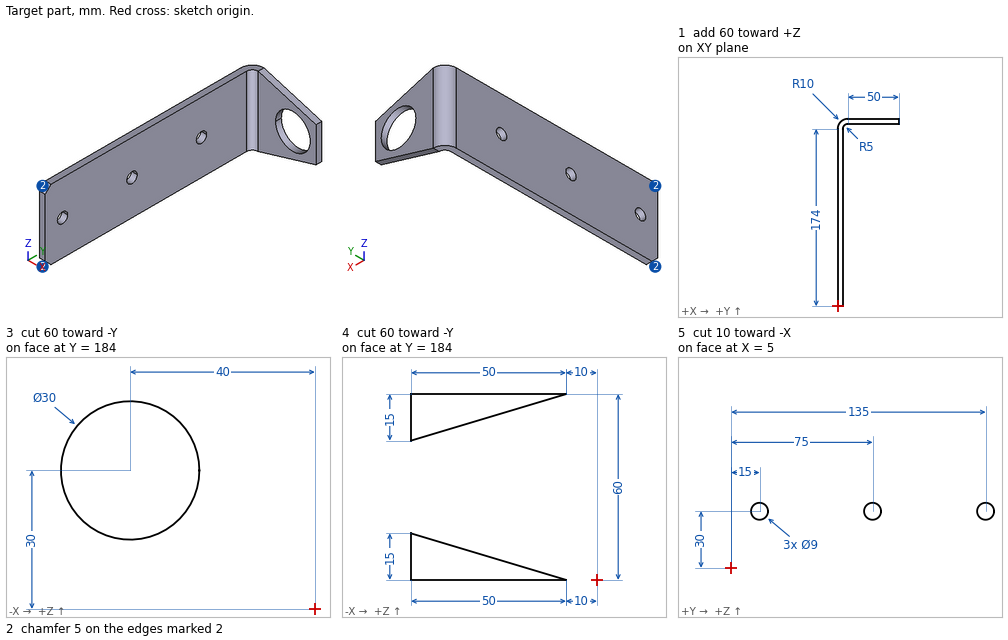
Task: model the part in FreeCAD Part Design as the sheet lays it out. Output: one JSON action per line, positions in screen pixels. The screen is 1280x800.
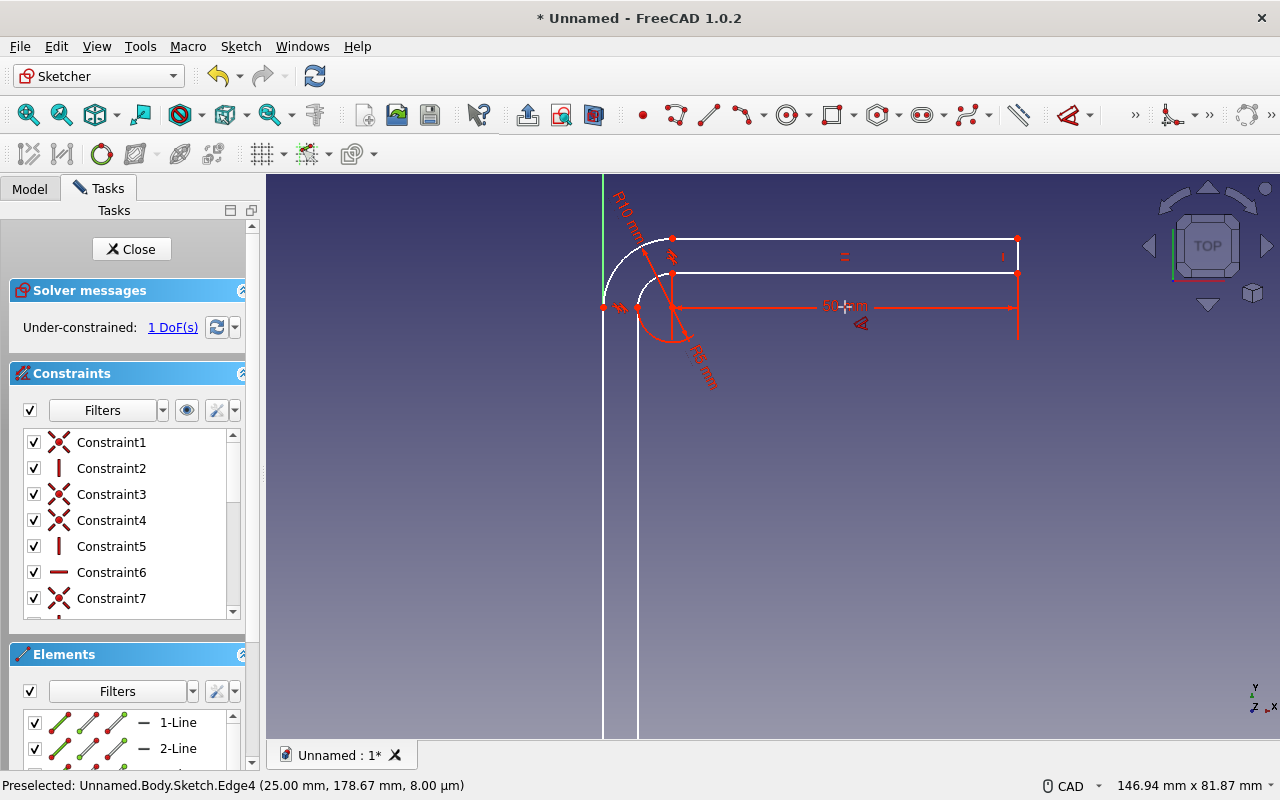
{"action": "left_click", "coordinate": [603, 668]}
{"action": "left_click", "coordinate": [569, 509]}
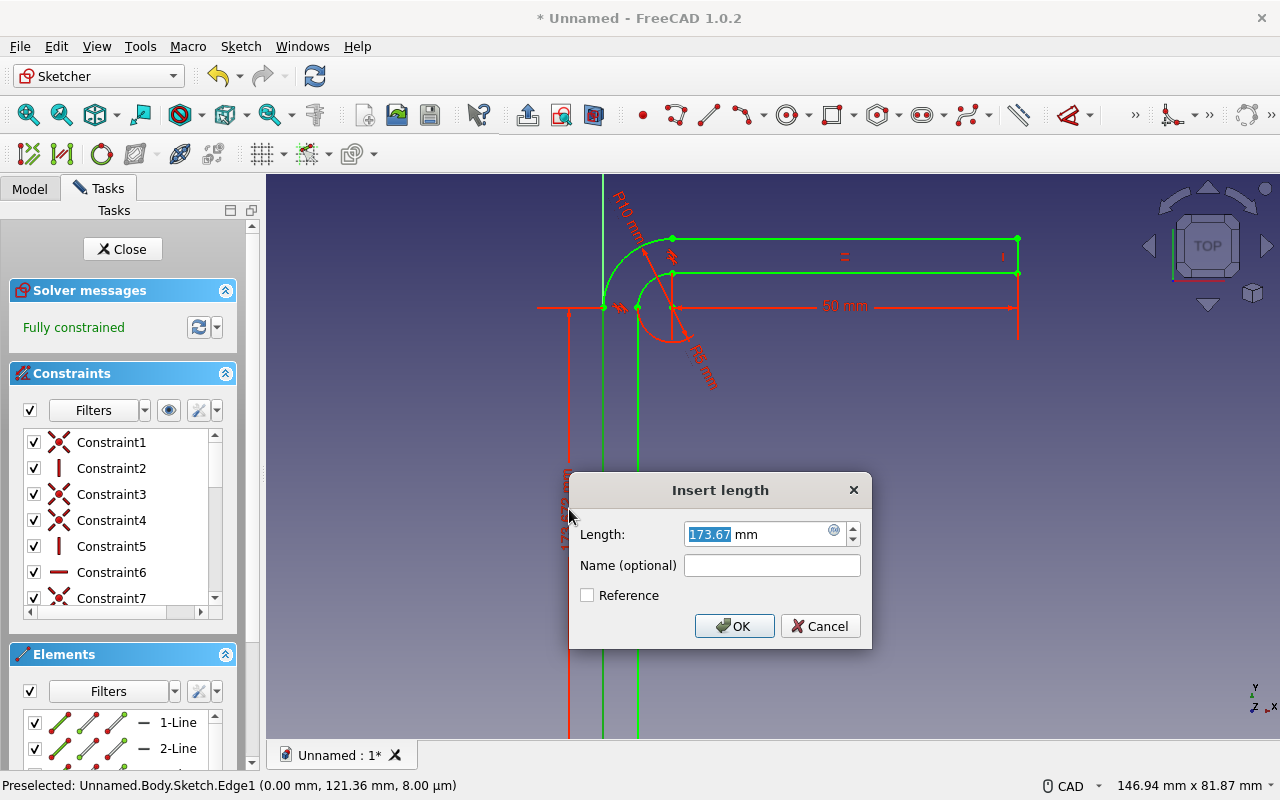
{"action": "type", "text": "174"}
{"action": "key", "text": "Return"}
{"action": "key", "text": "Escape"}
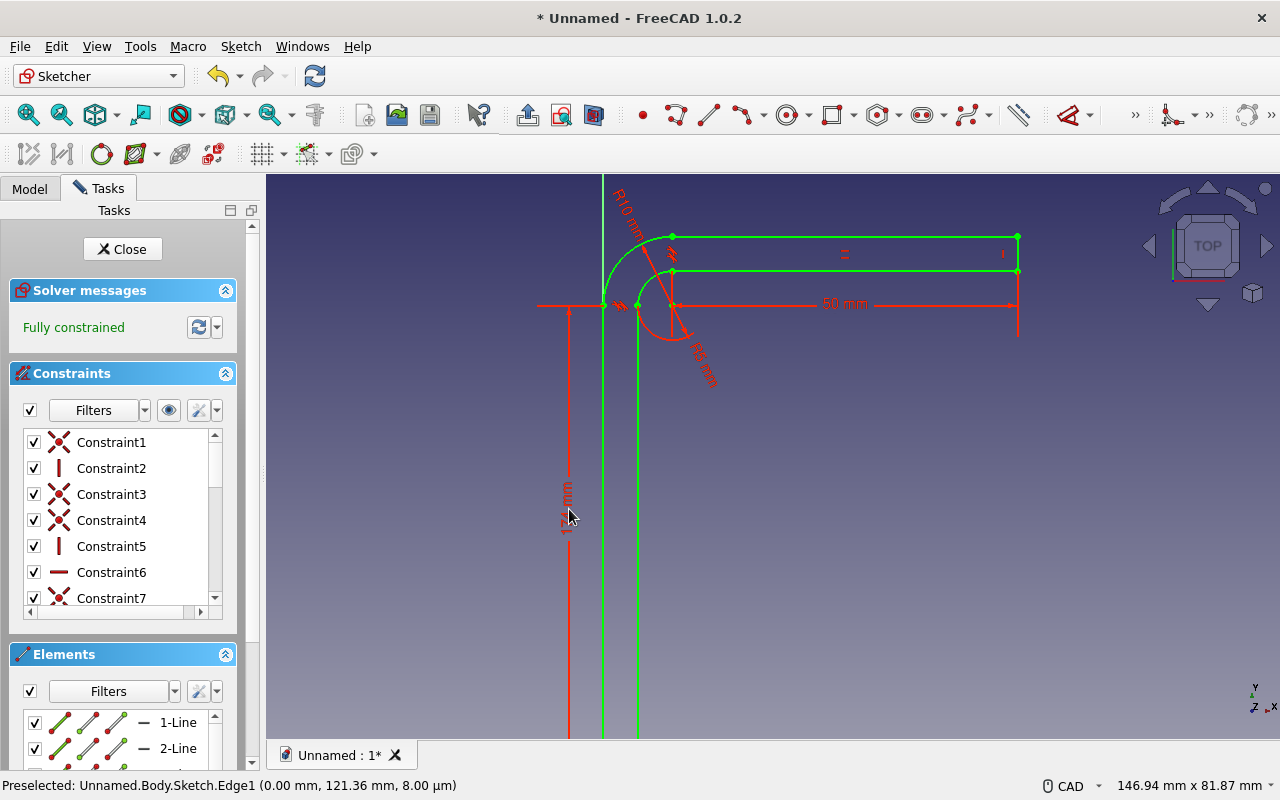
{"action": "left_click", "coordinate": [123, 249]}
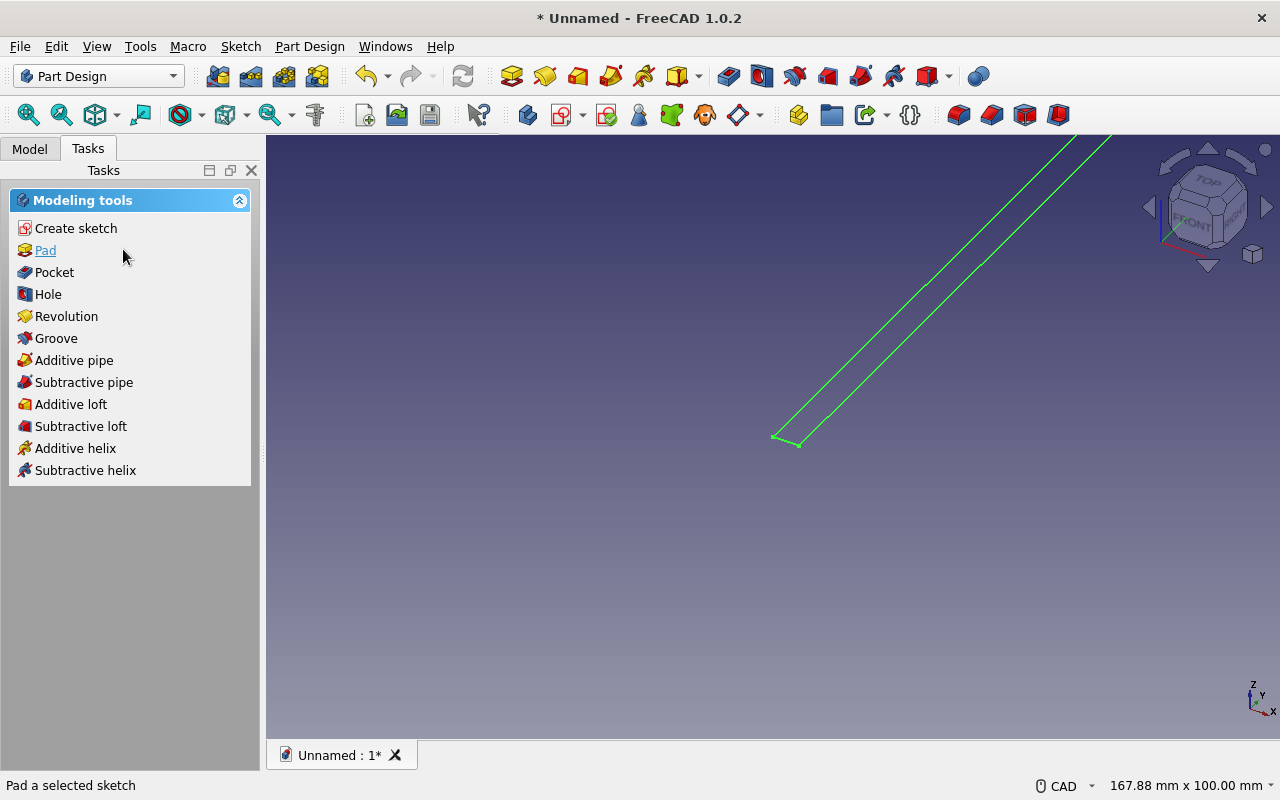
{"action": "left_click", "coordinate": [512, 76]}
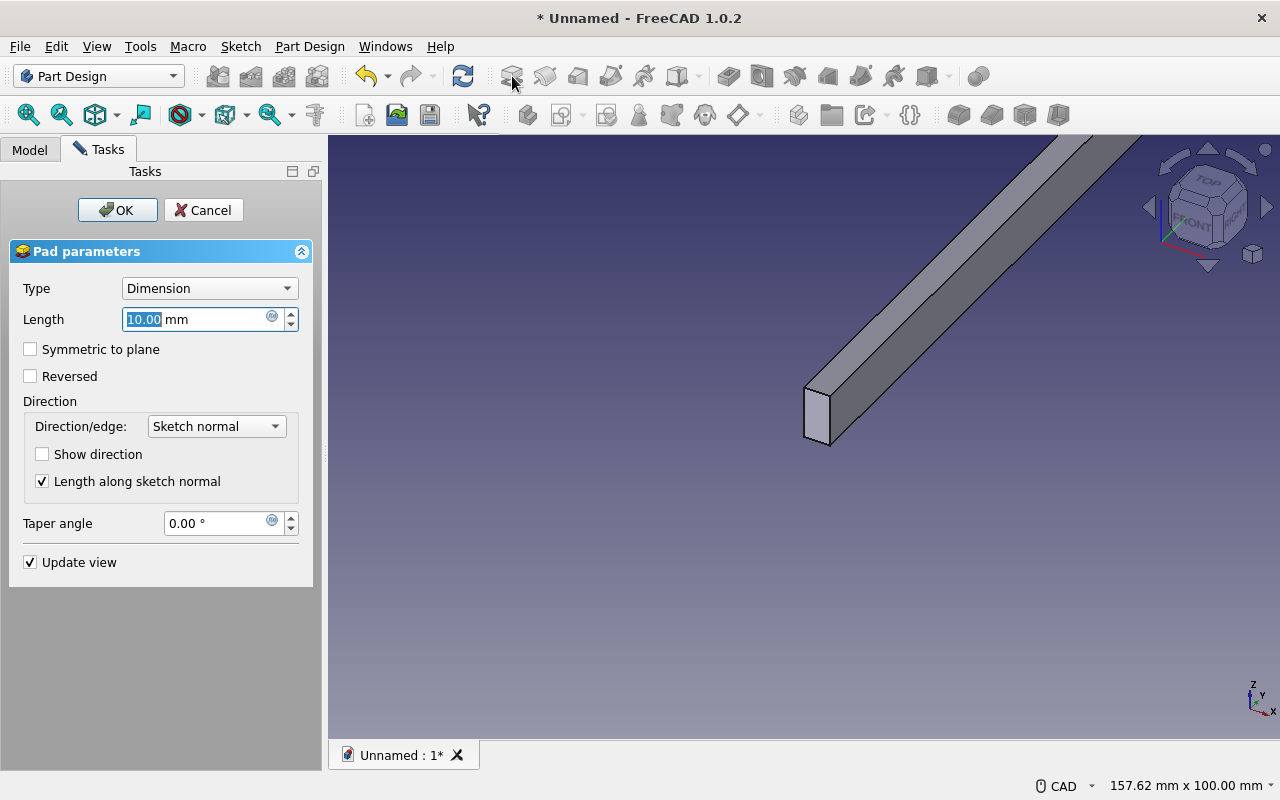
{"action": "type", "text": "60"}
{"action": "key", "text": "Tab"}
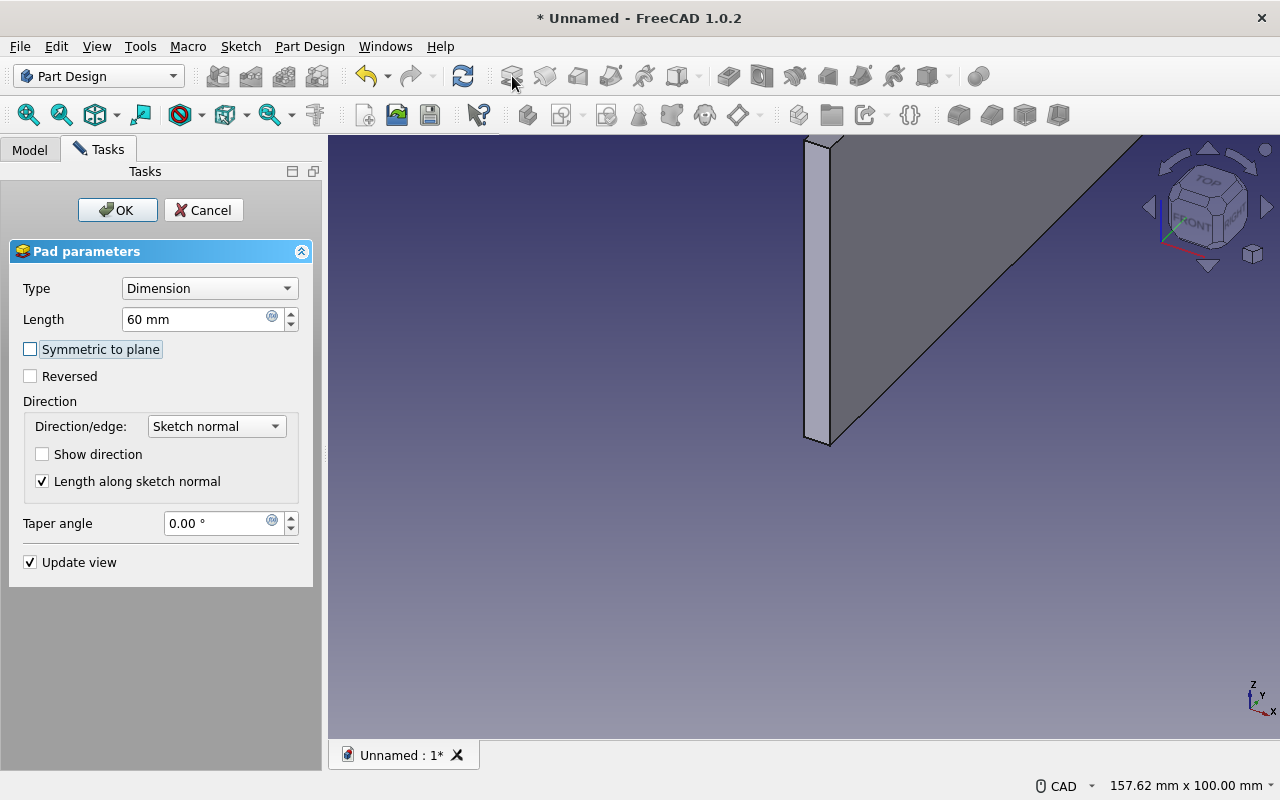
{"action": "left_click", "coordinate": [118, 210]}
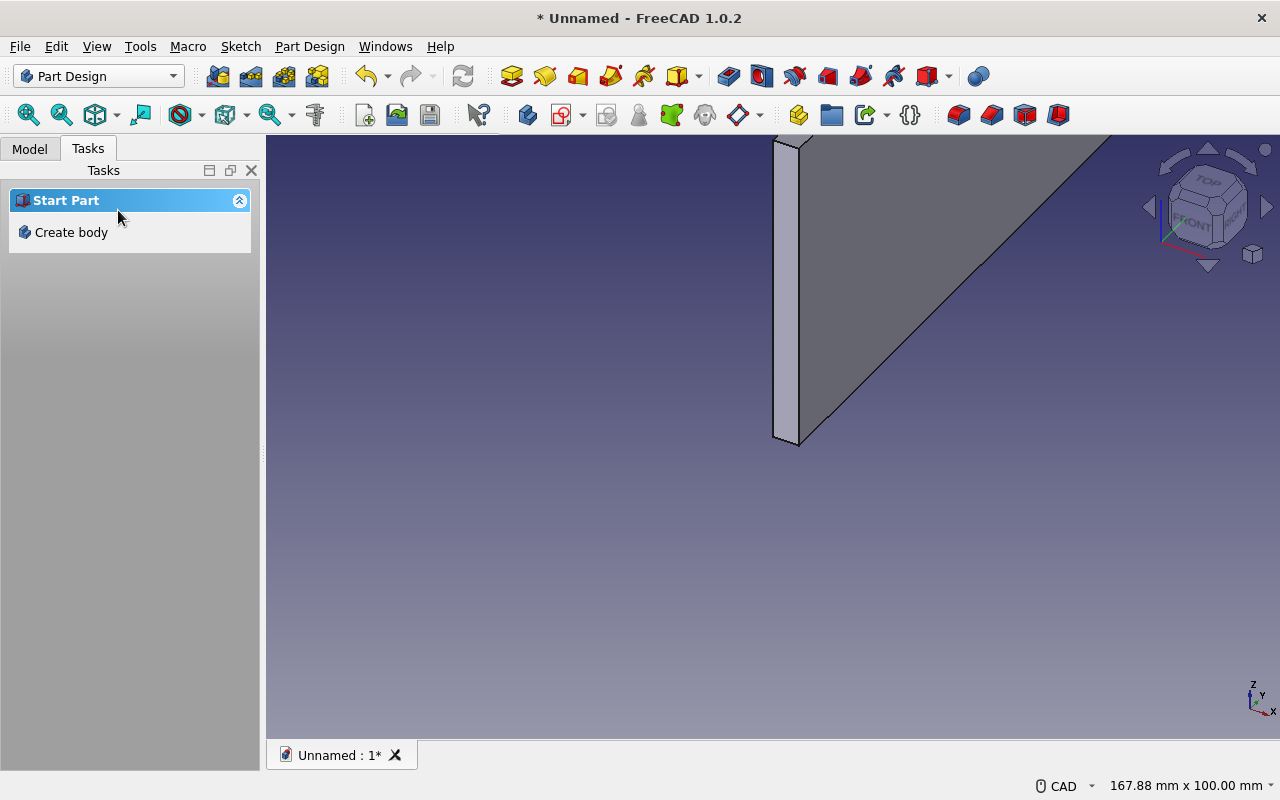
{"action": "key", "text": "v f"}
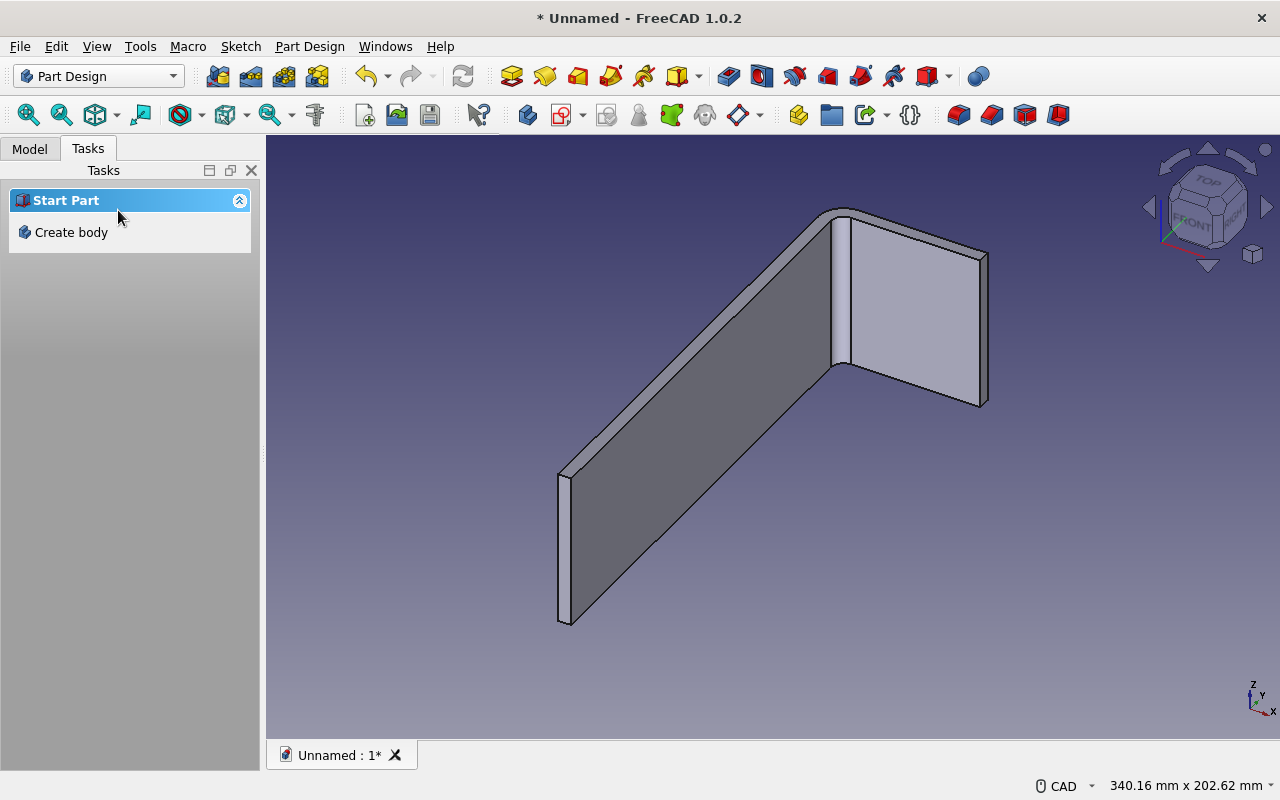
{"action": "left_click", "coordinate": [565, 475]}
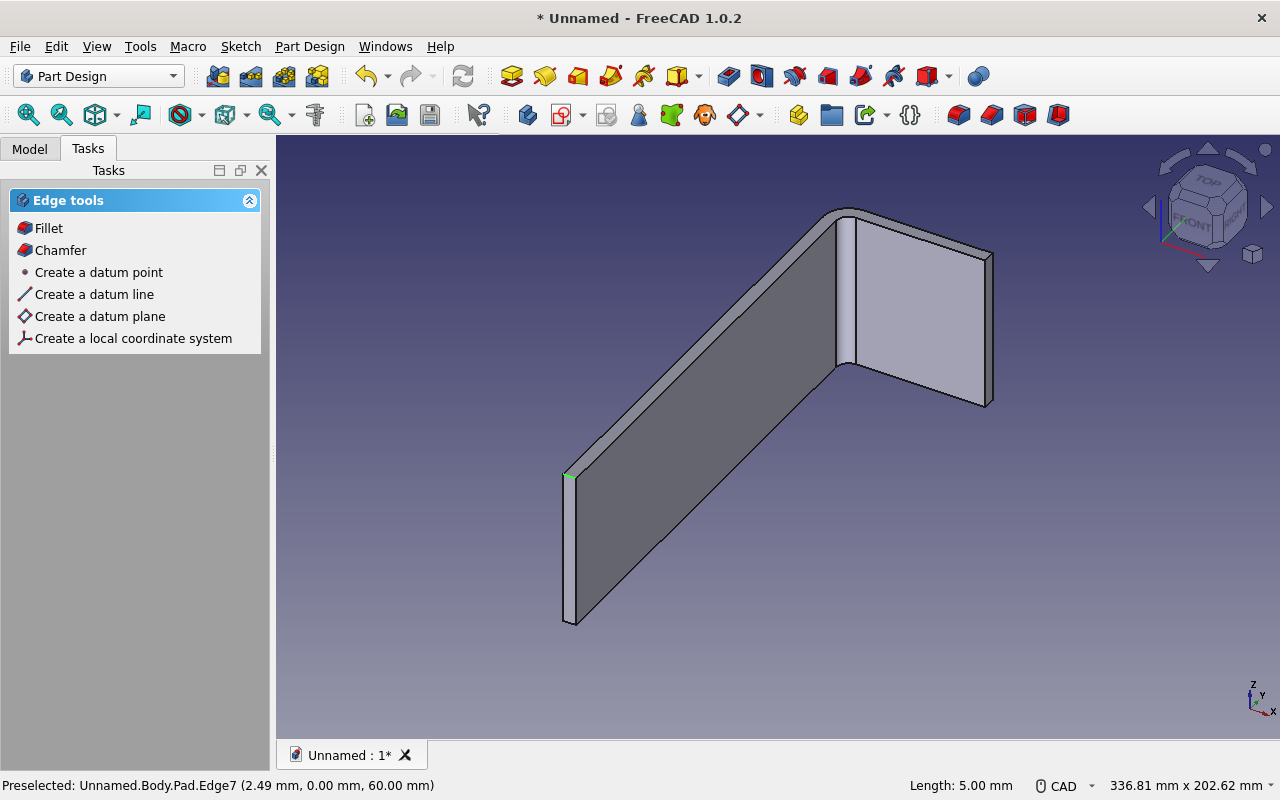
{"action": "scroll", "coordinate": [570, 622], "scroll_direction": "up", "scroll_amount": 5}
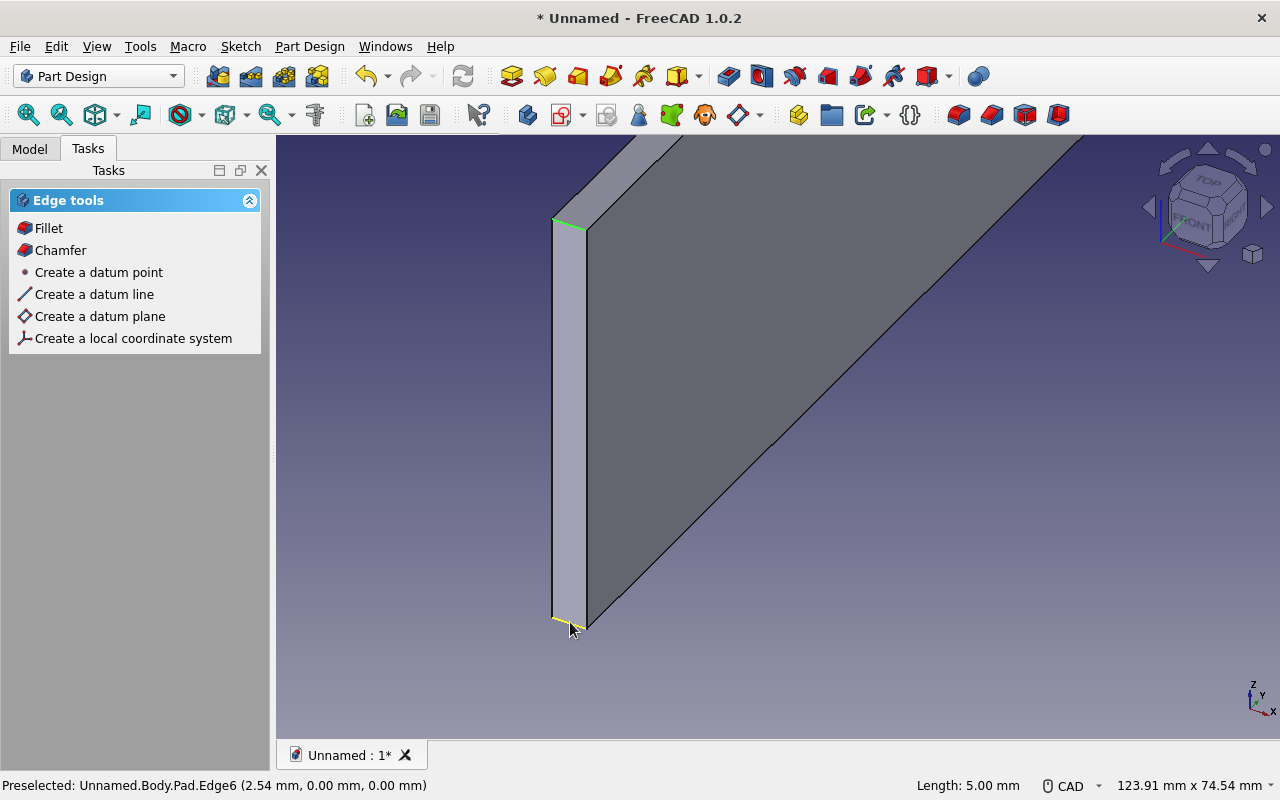
{"action": "left_click", "coordinate": [29, 116]}